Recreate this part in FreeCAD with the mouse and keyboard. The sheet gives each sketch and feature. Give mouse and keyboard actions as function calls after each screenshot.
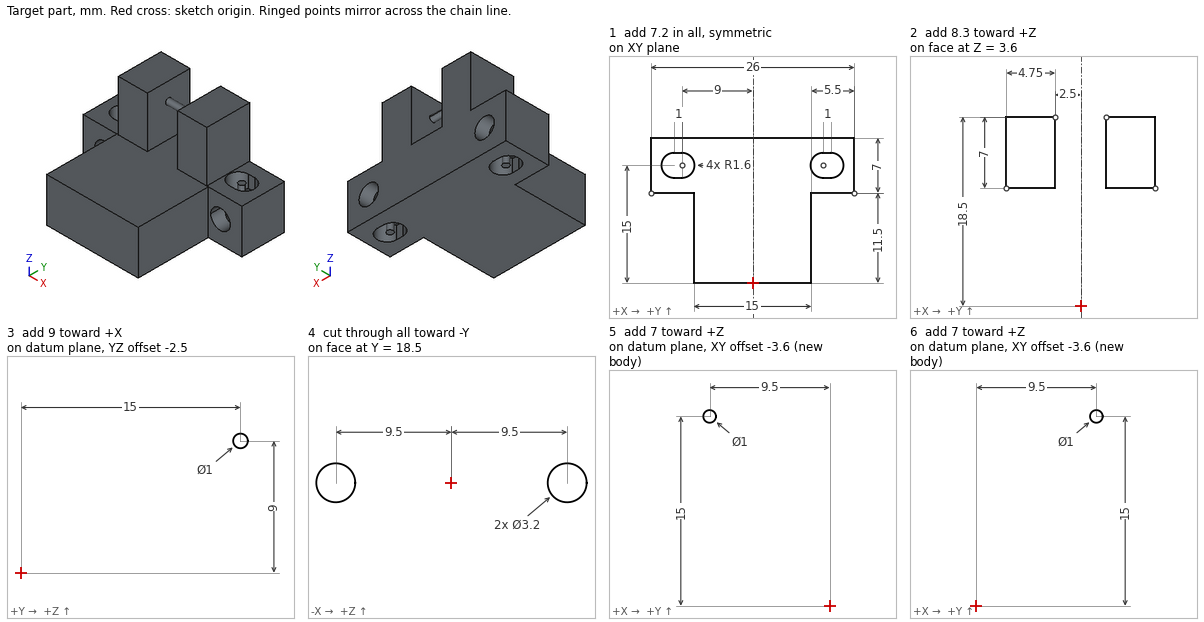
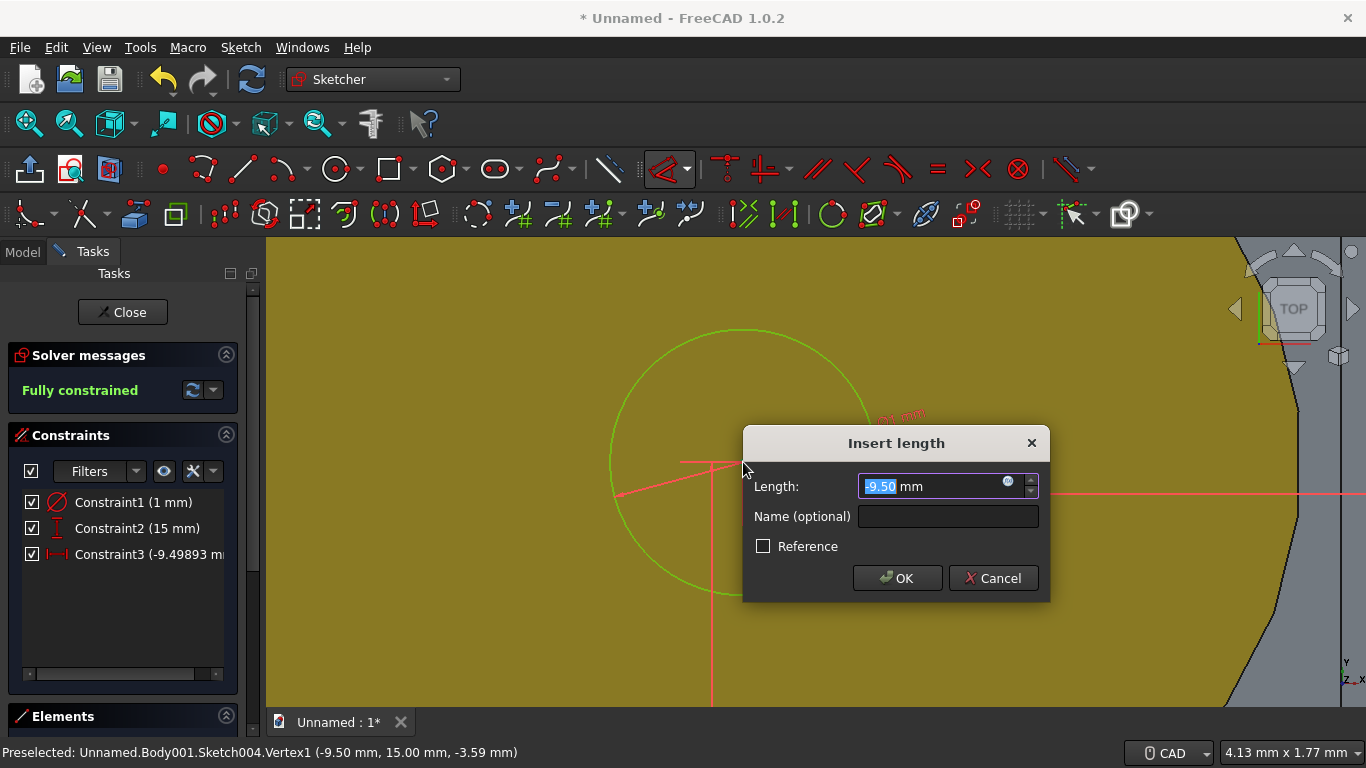
text(-9.5)
key(Return)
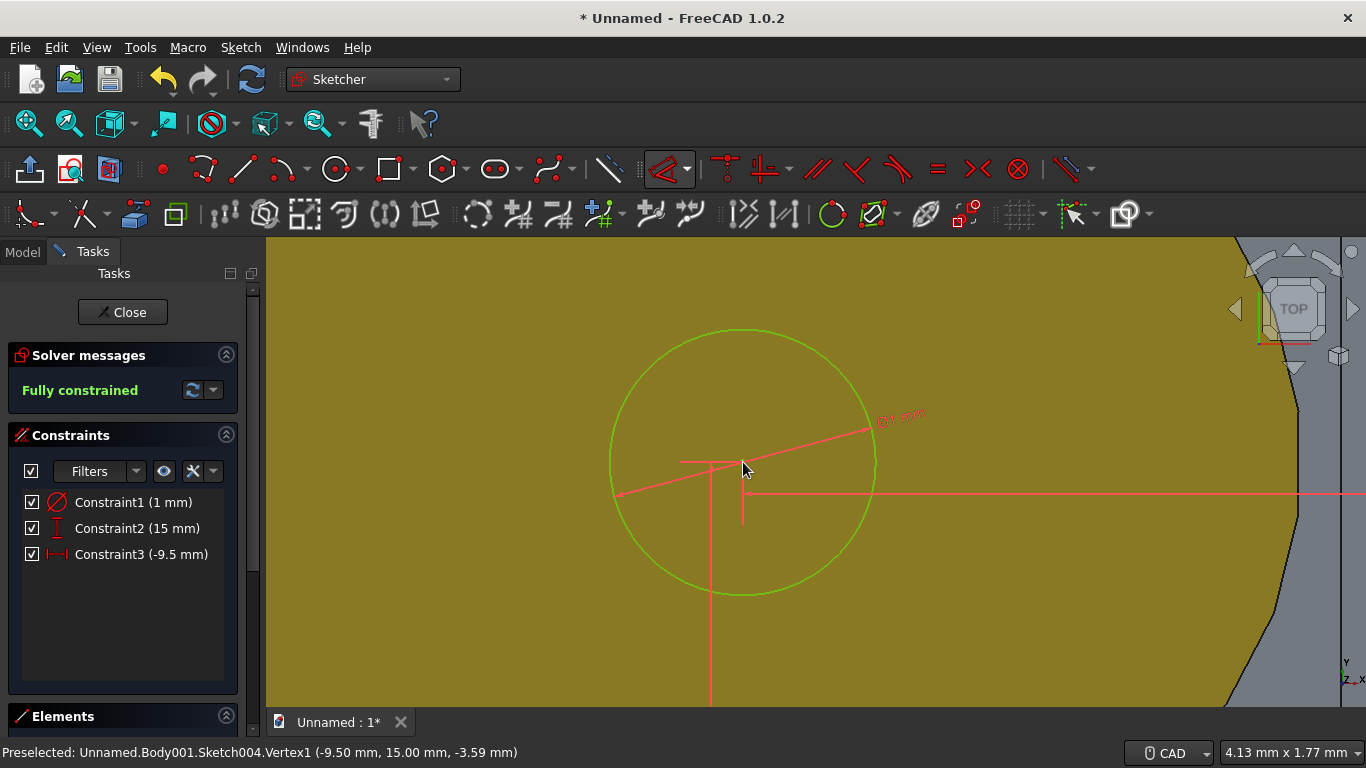
click(123, 312)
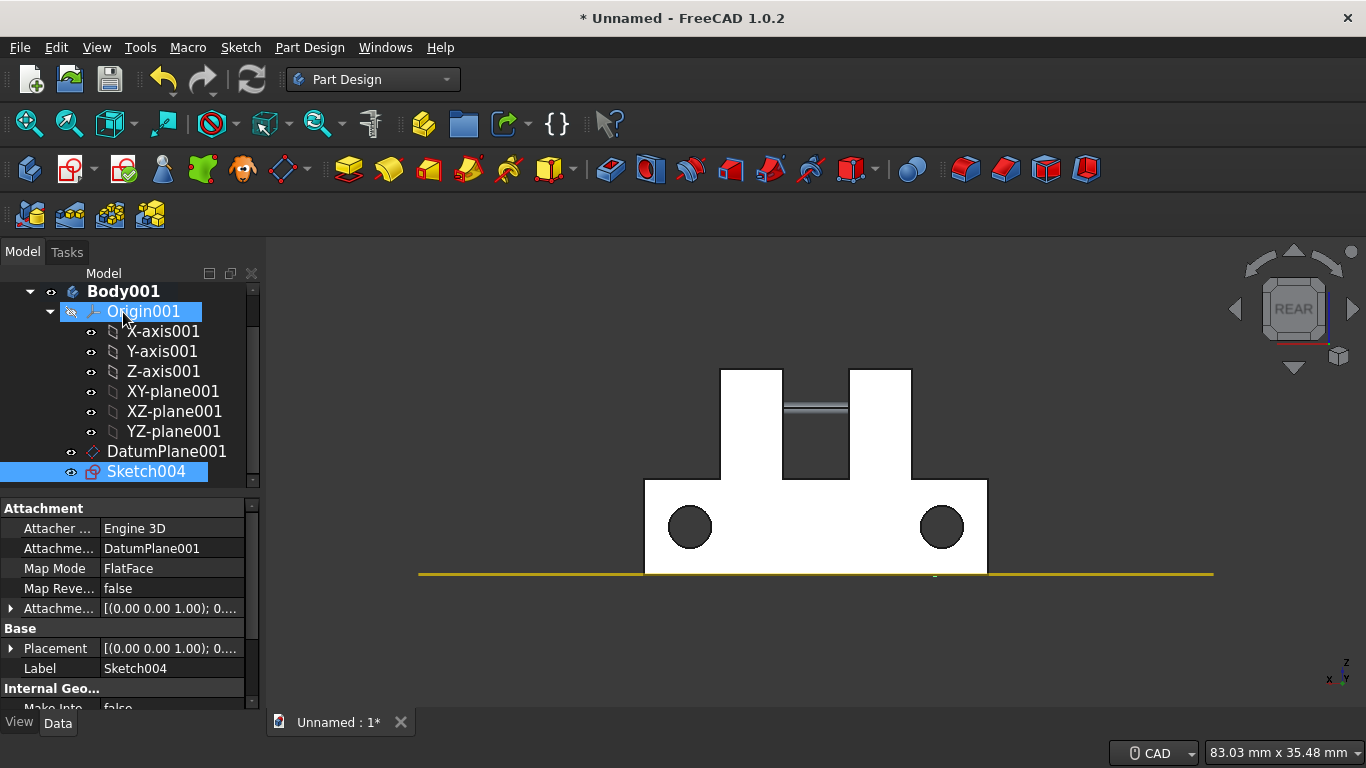
click(350, 170)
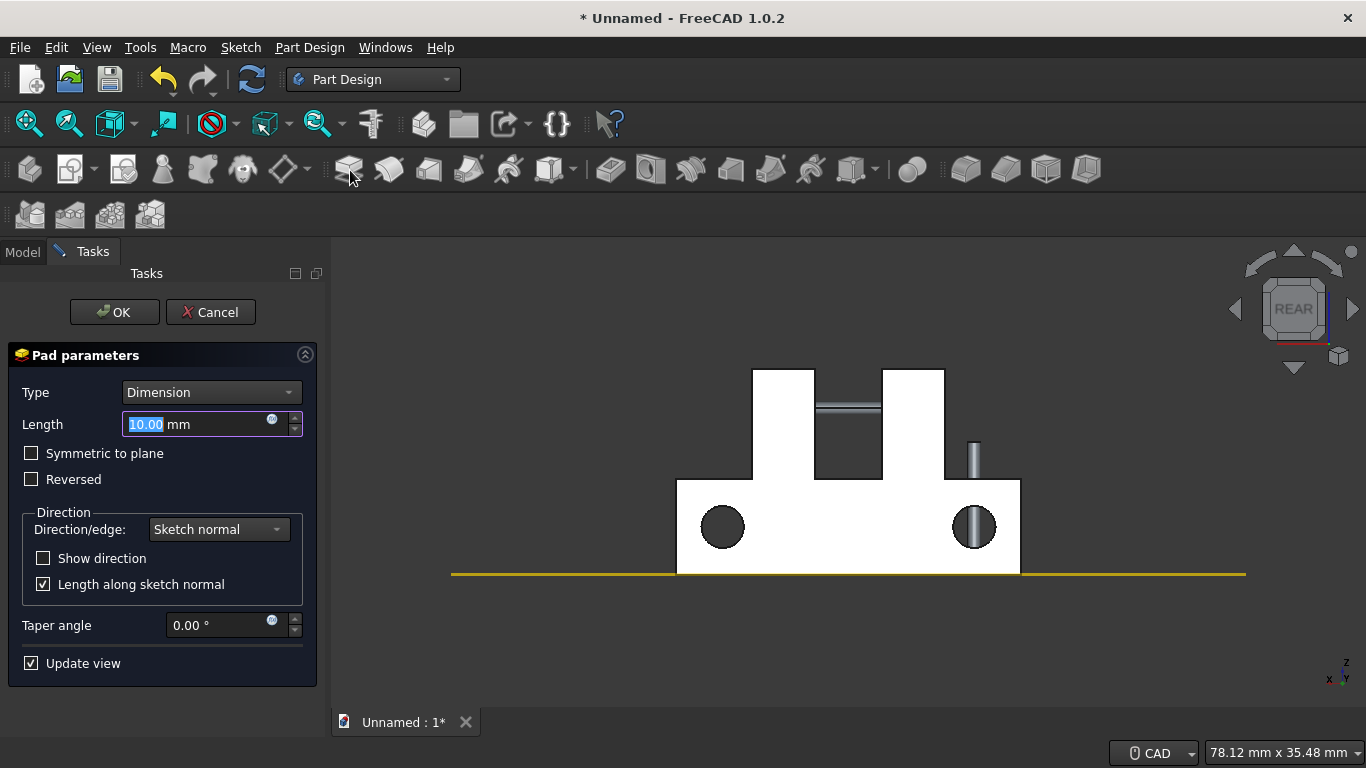
text(7)
key(Tab)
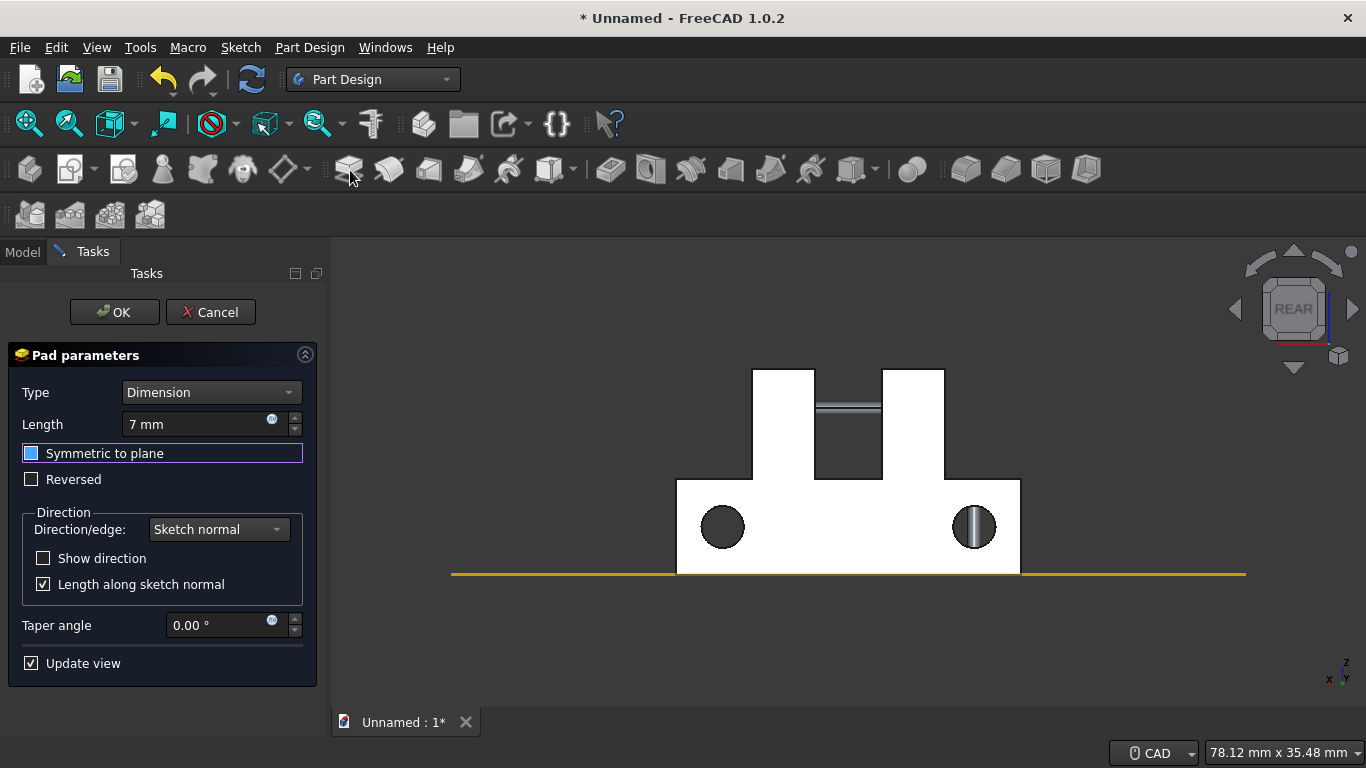
click(115, 312)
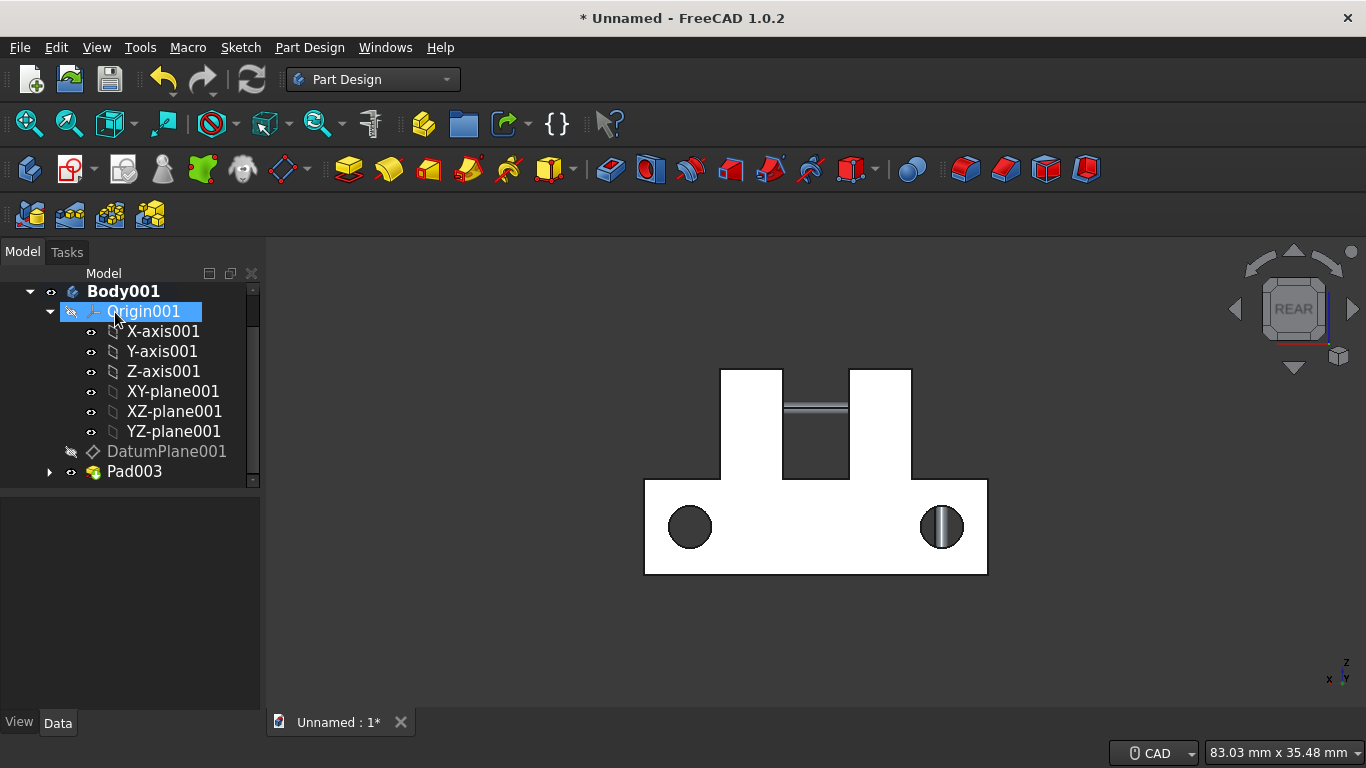
click(30, 124)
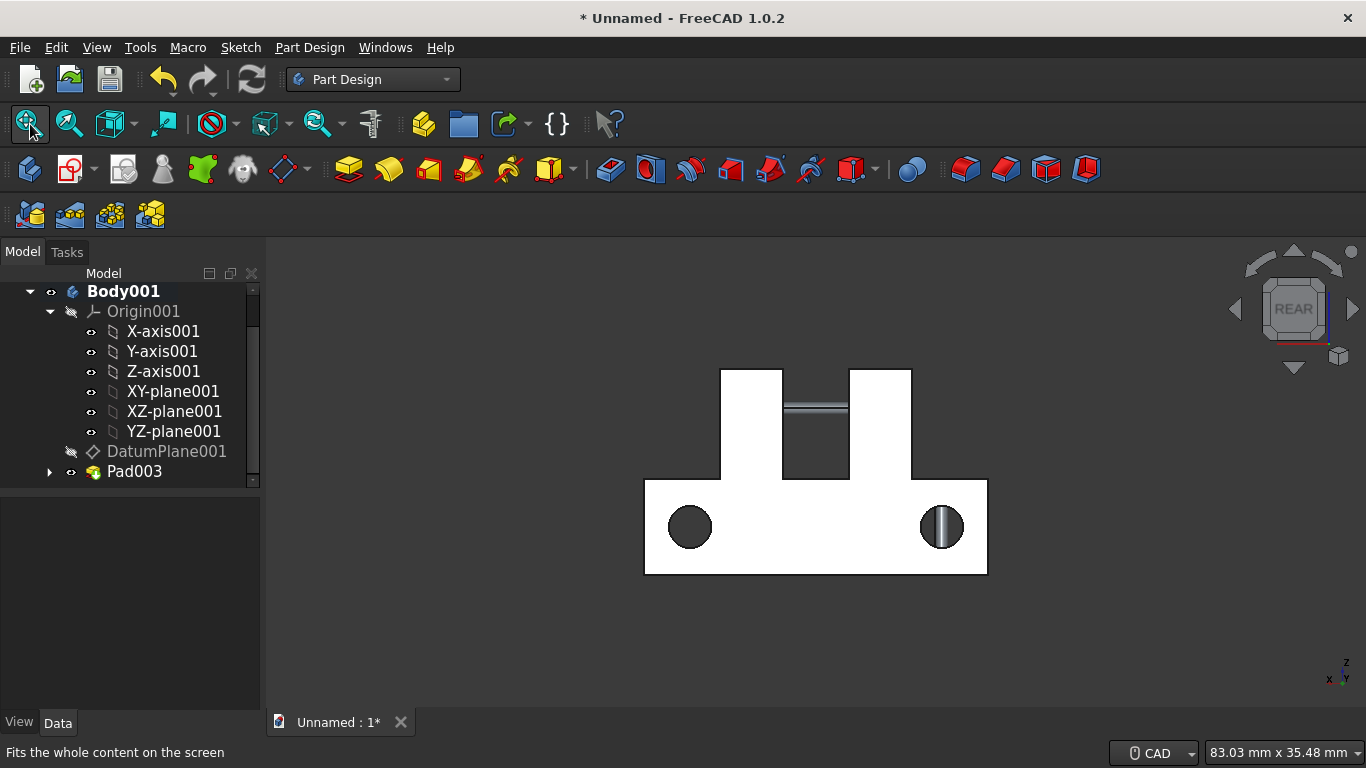
click(30, 170)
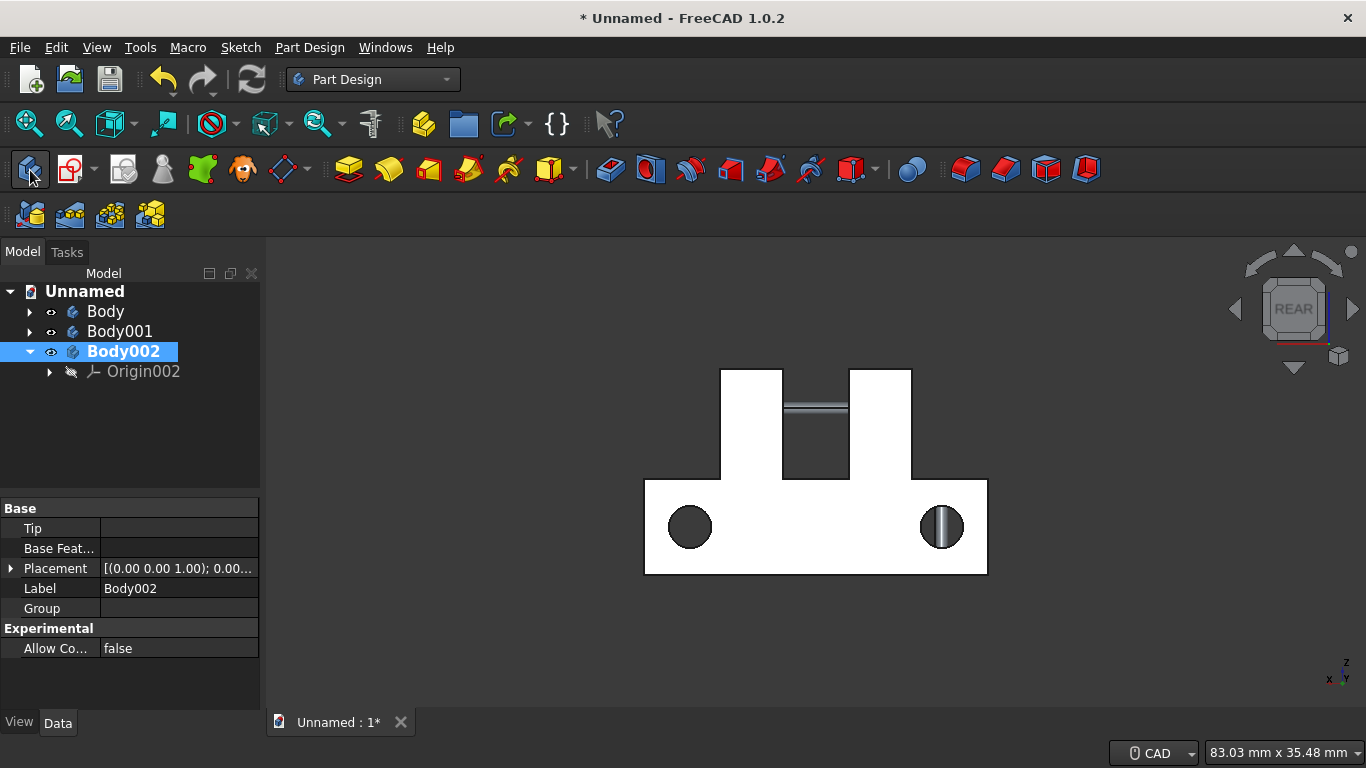
click(50, 372)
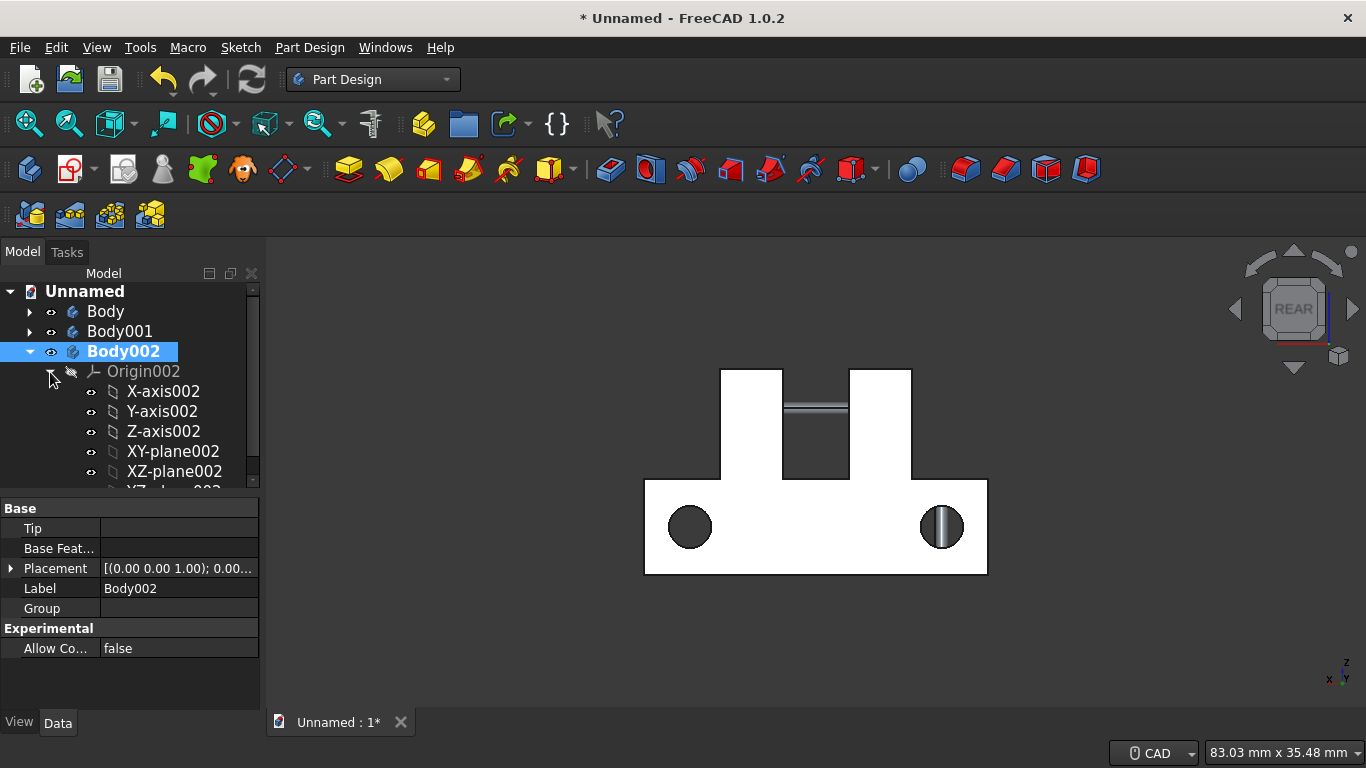
click(136, 452)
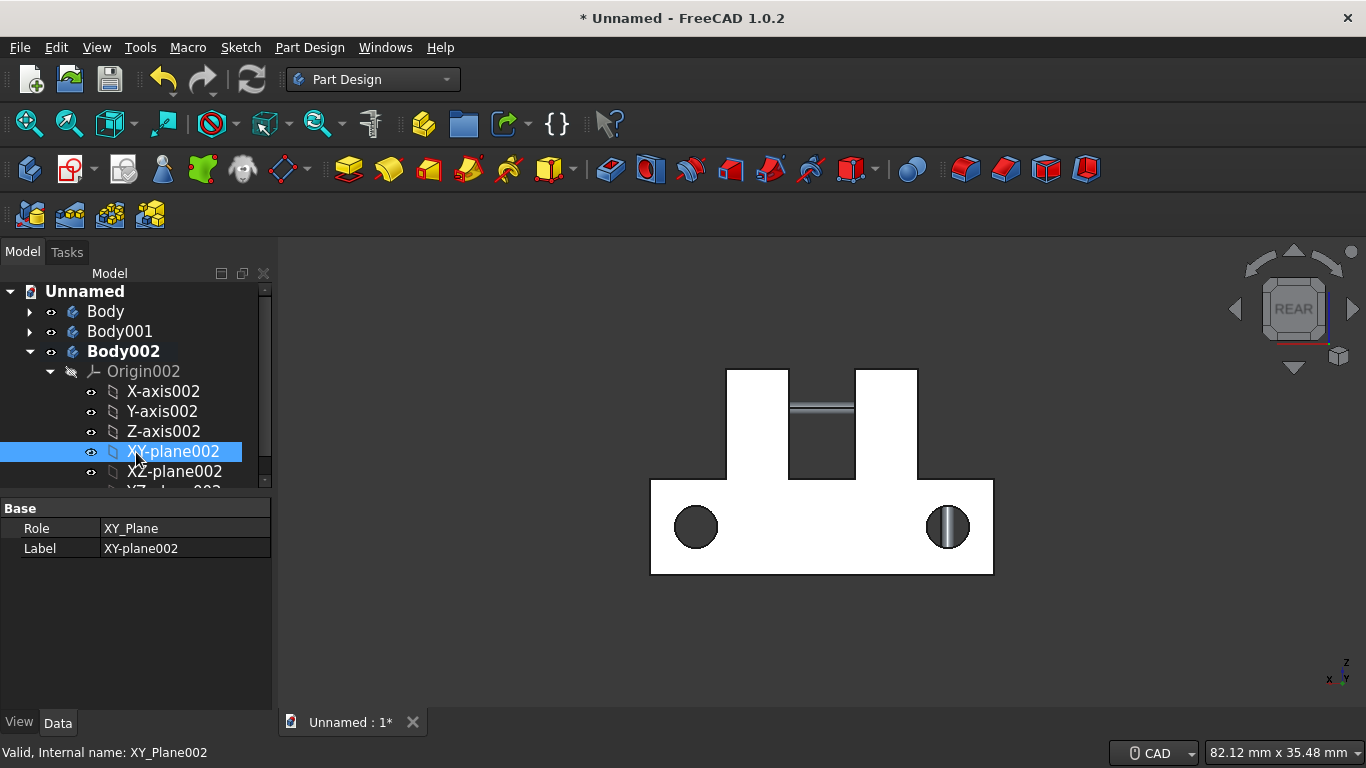
click(284, 170)